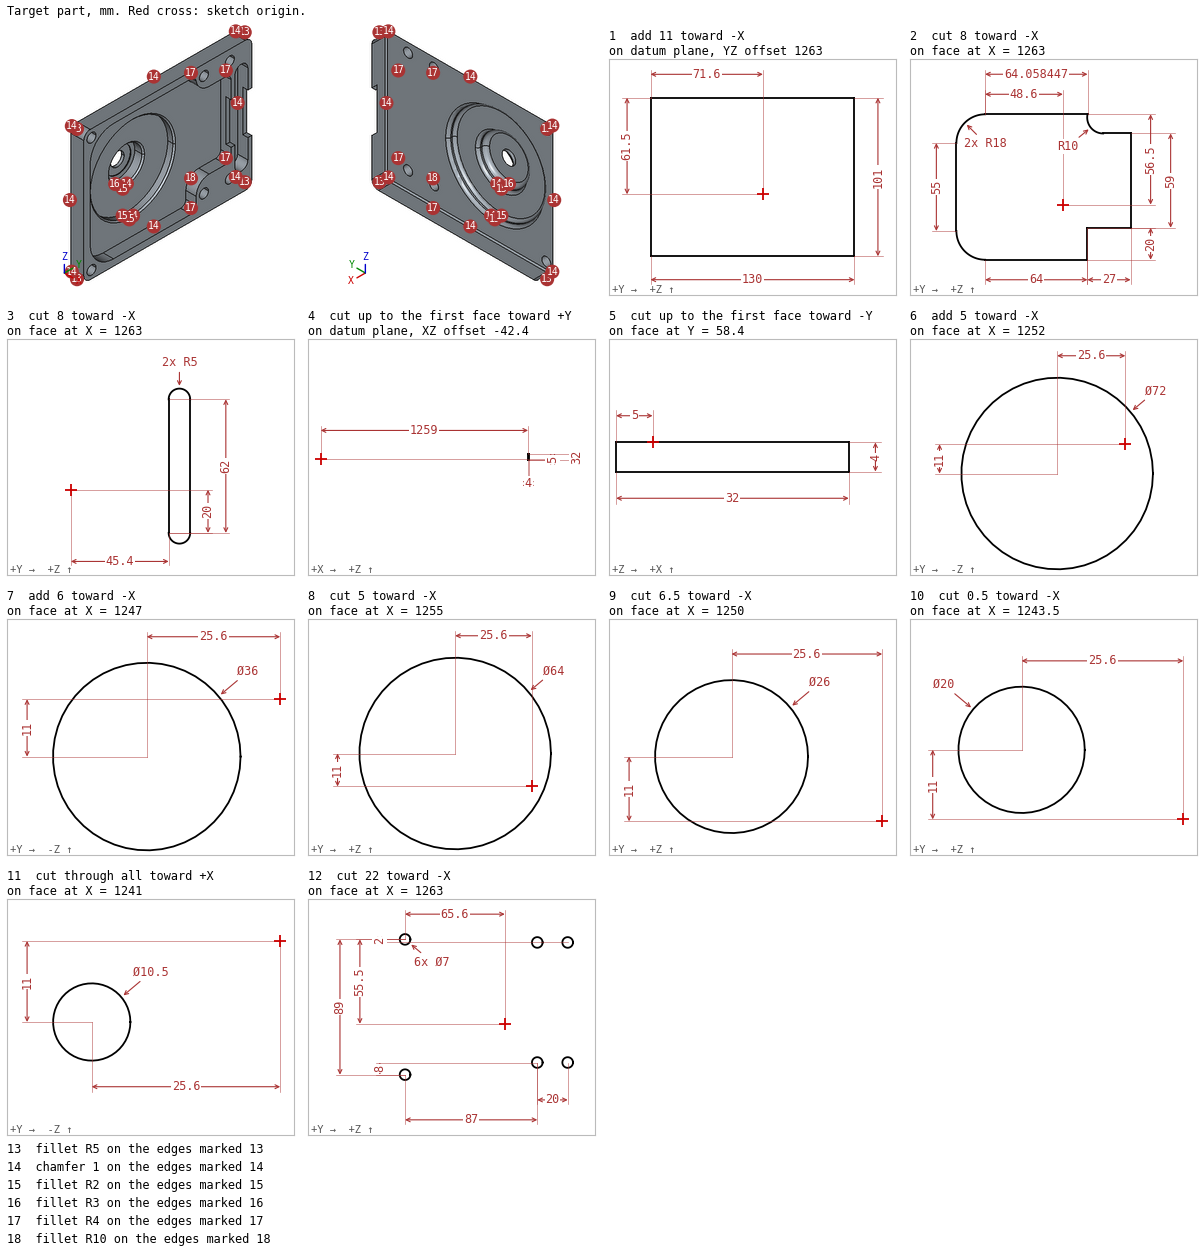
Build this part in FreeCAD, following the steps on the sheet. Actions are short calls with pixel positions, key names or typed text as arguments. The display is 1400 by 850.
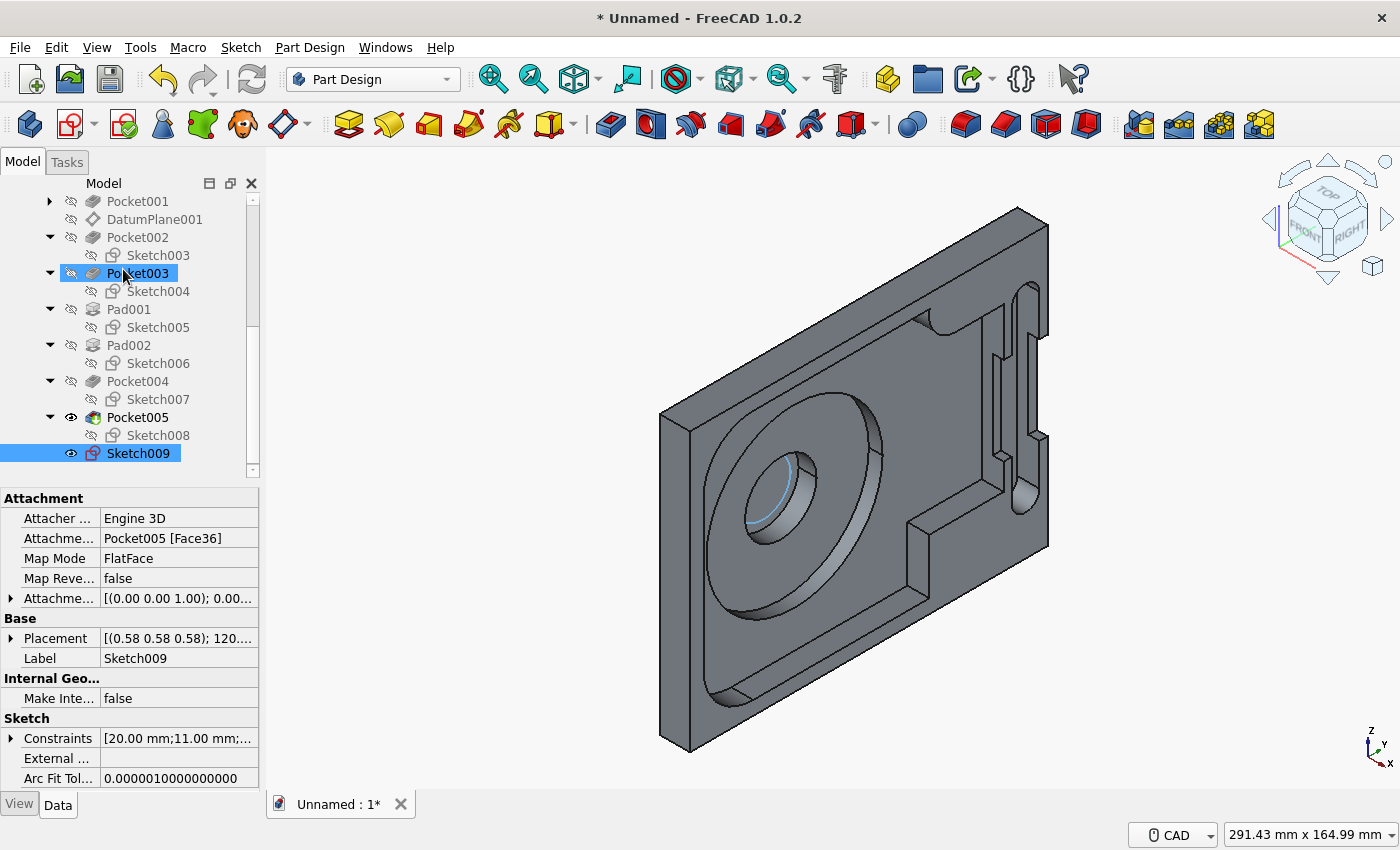
click(612, 124)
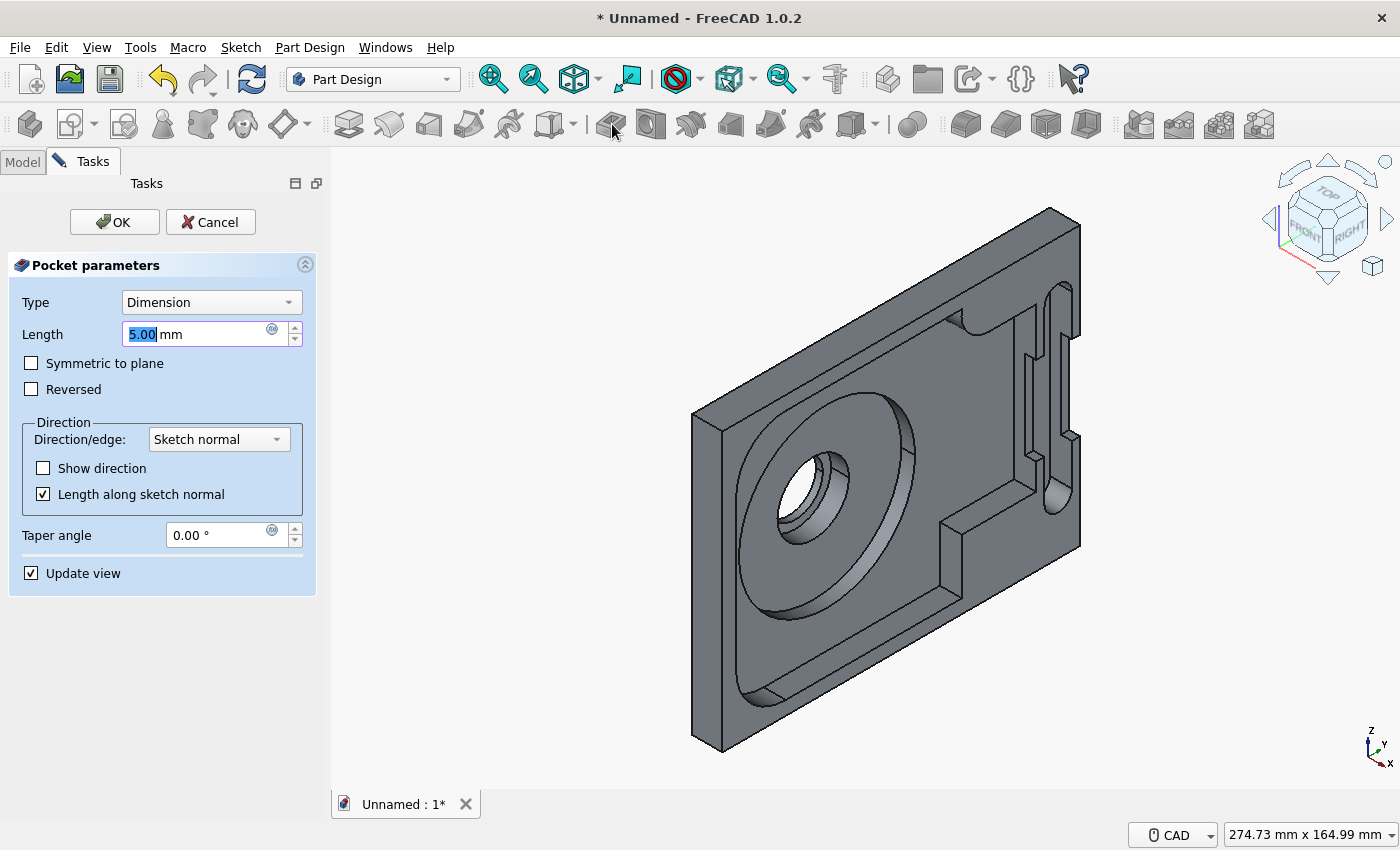
text(0.5)
key(Tab)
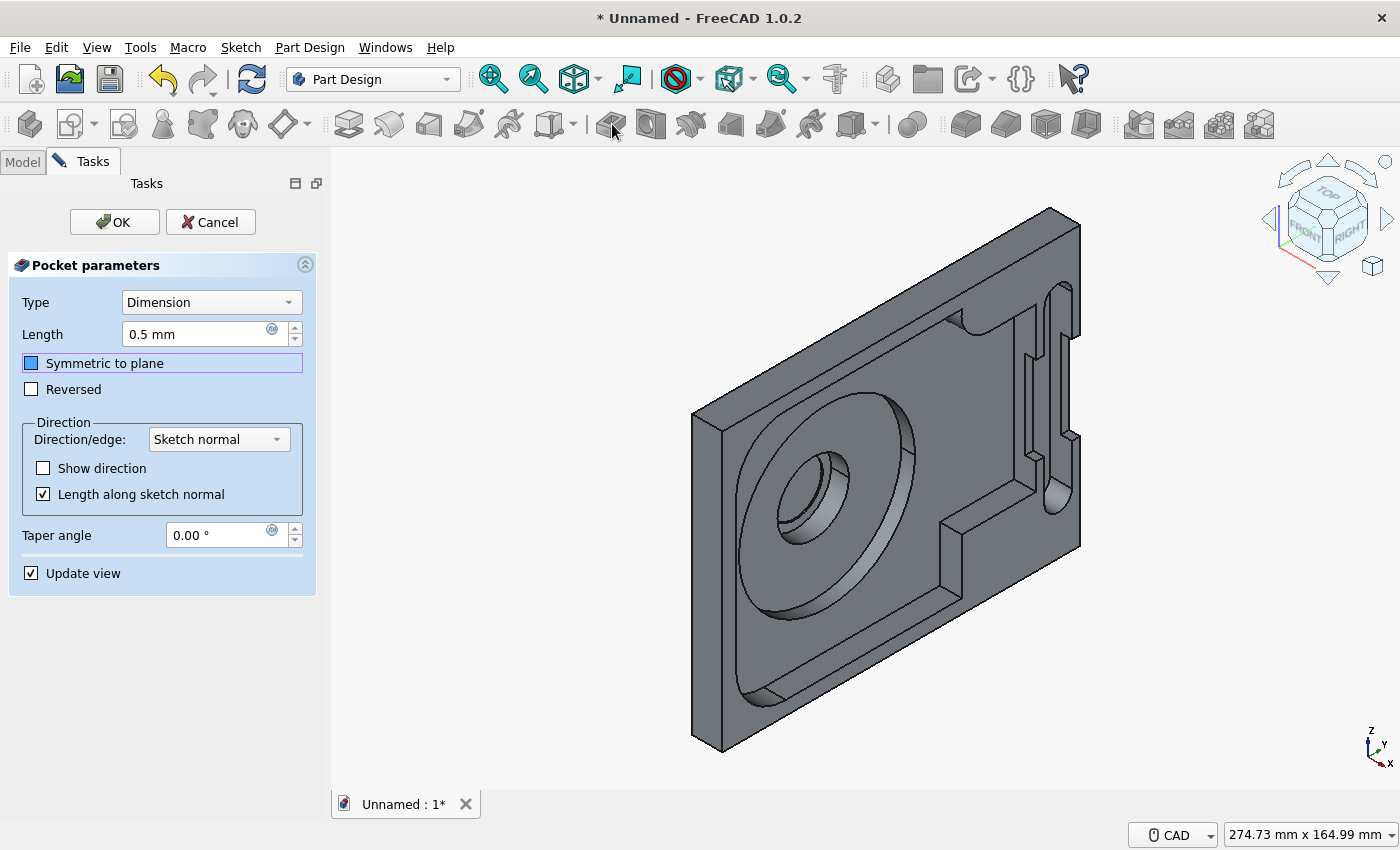
click(115, 222)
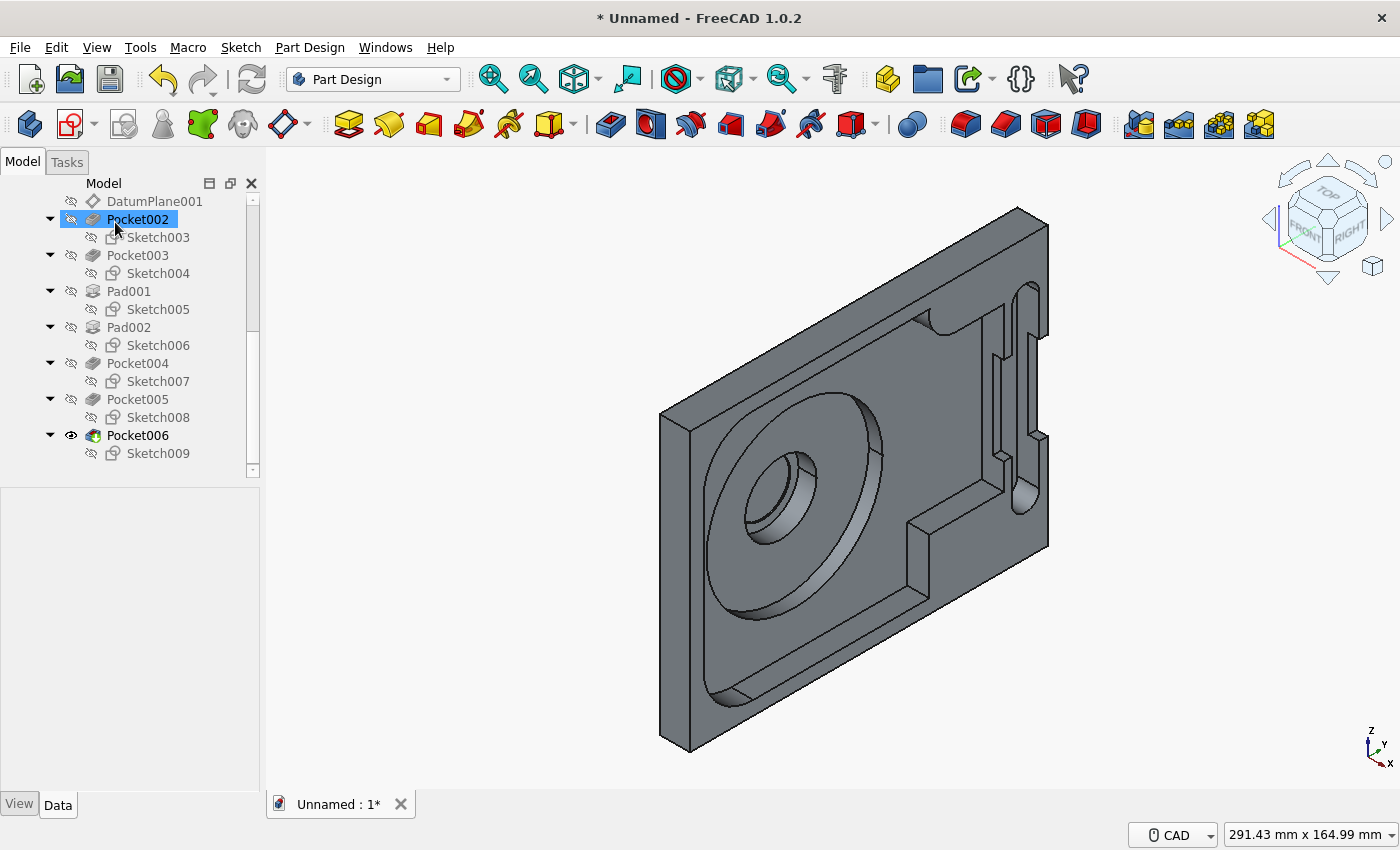
key(6)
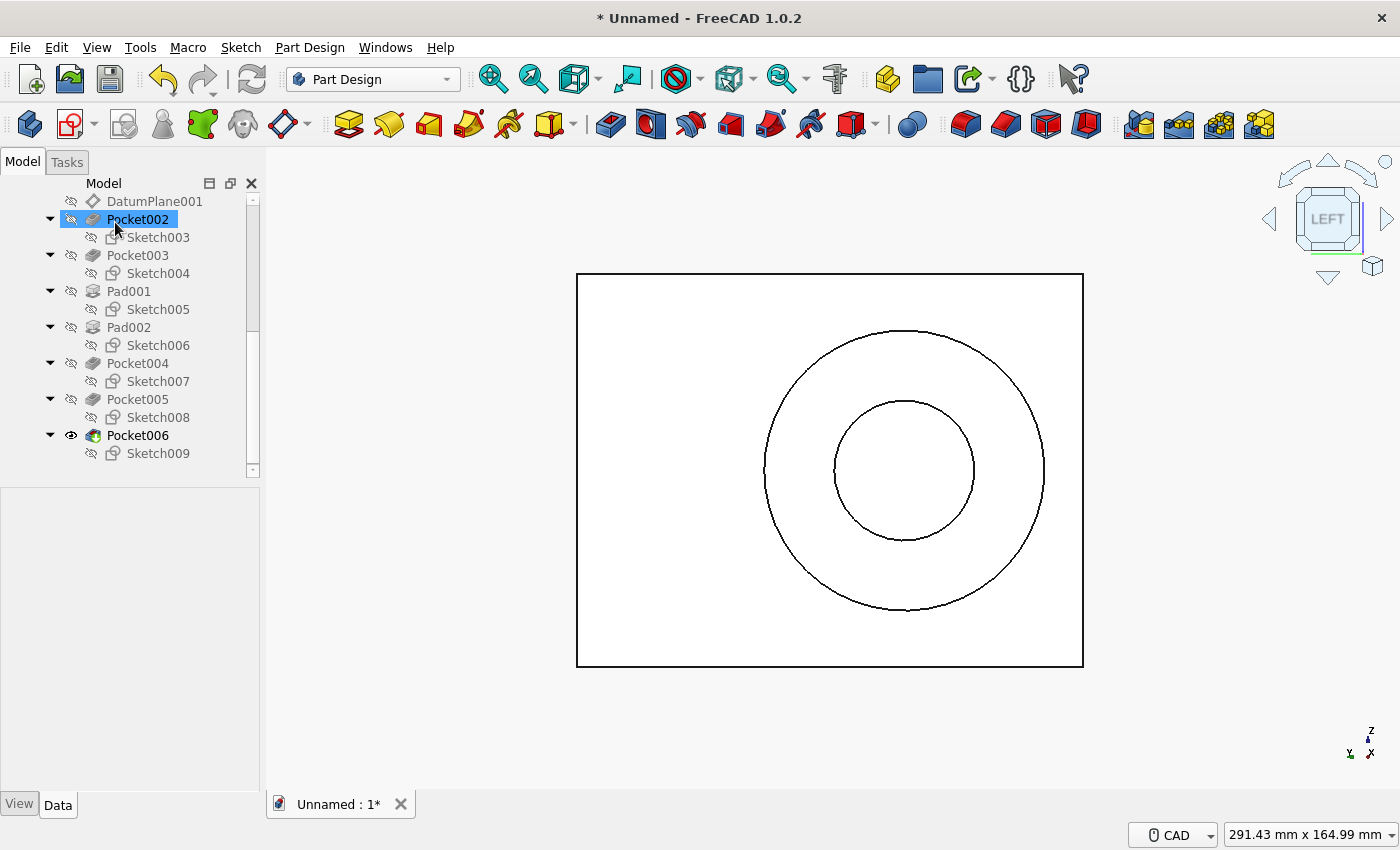
click(904, 470)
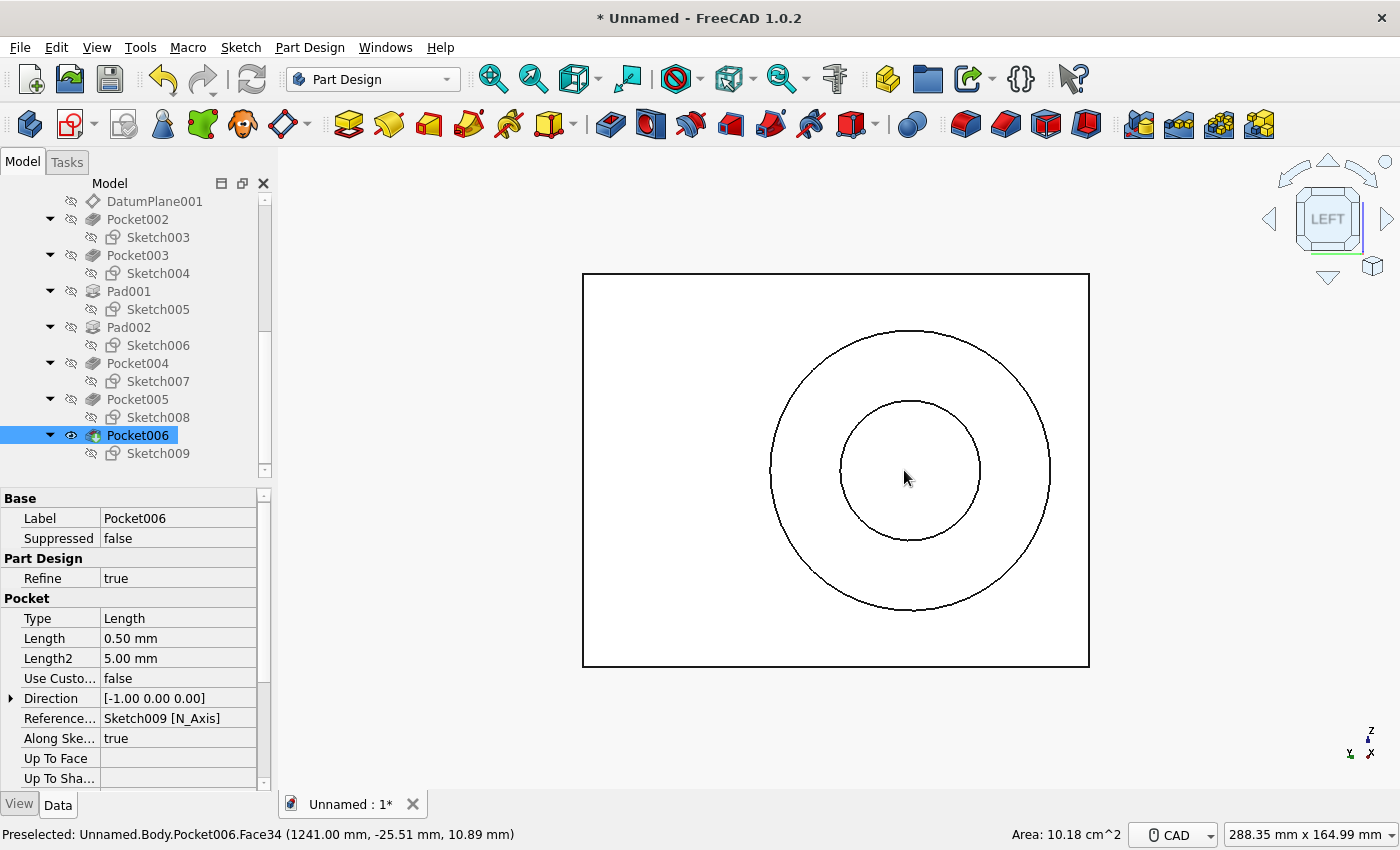
click(70, 124)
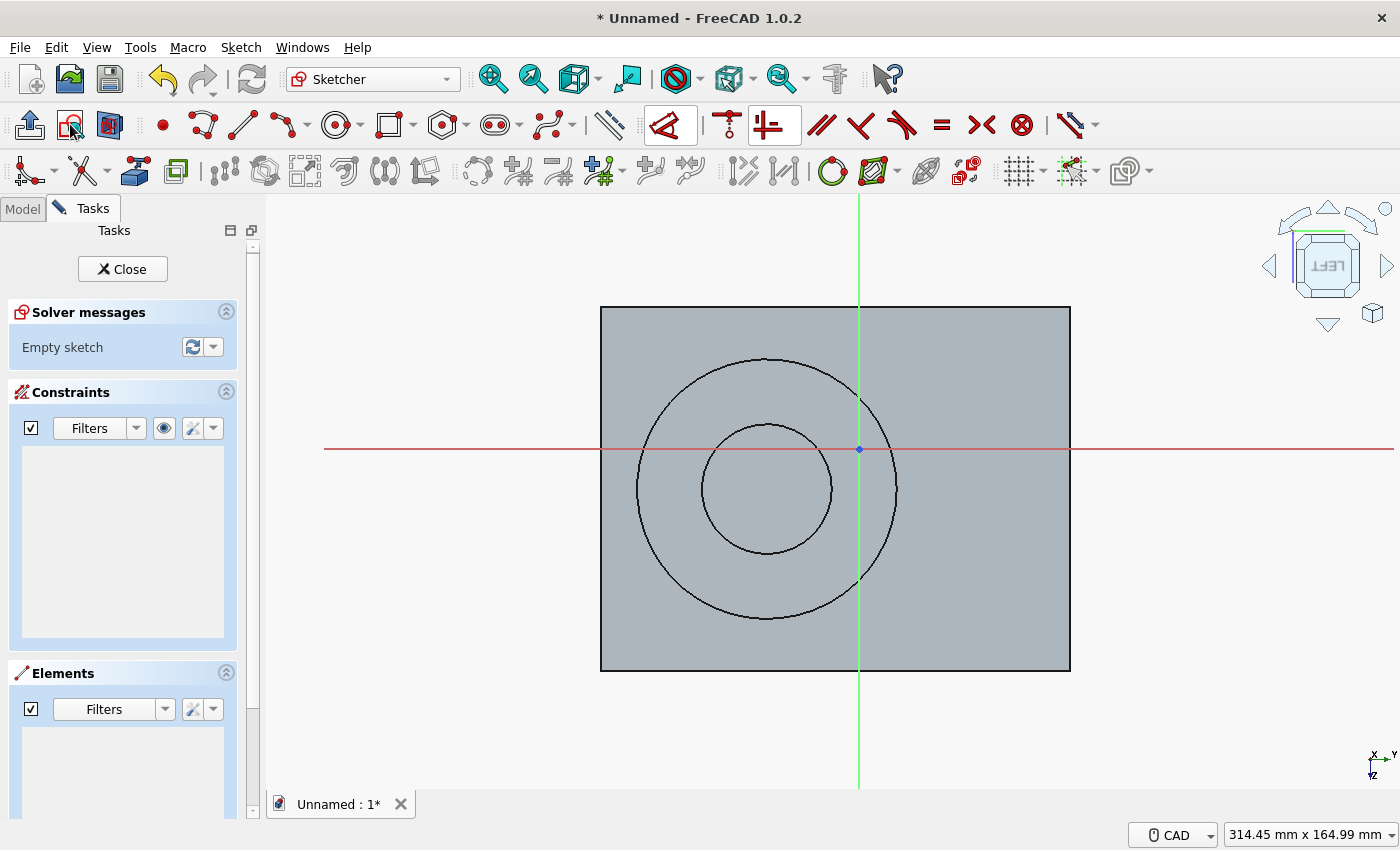
scroll(767, 489, up, 12)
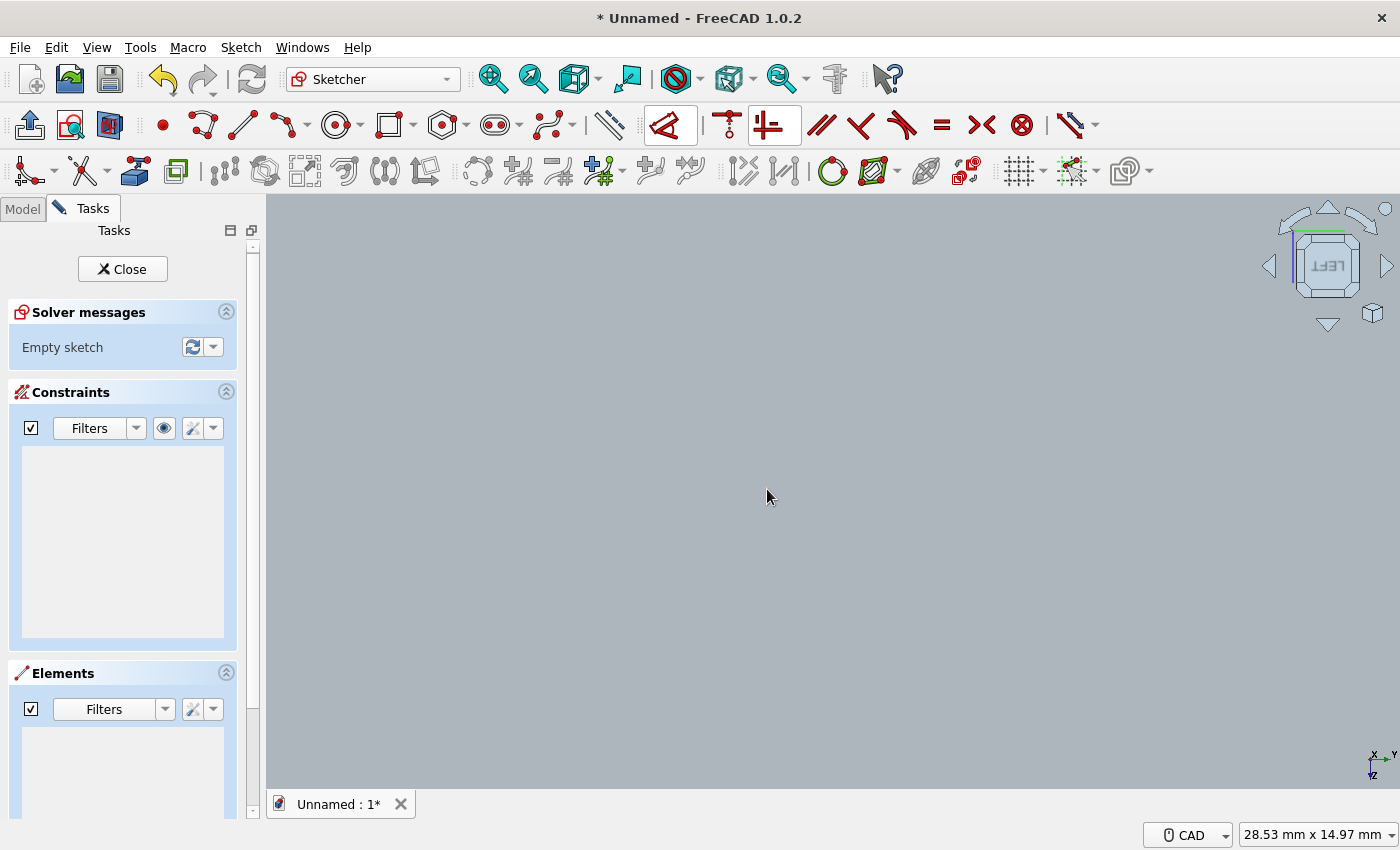
key(g)
key(c)